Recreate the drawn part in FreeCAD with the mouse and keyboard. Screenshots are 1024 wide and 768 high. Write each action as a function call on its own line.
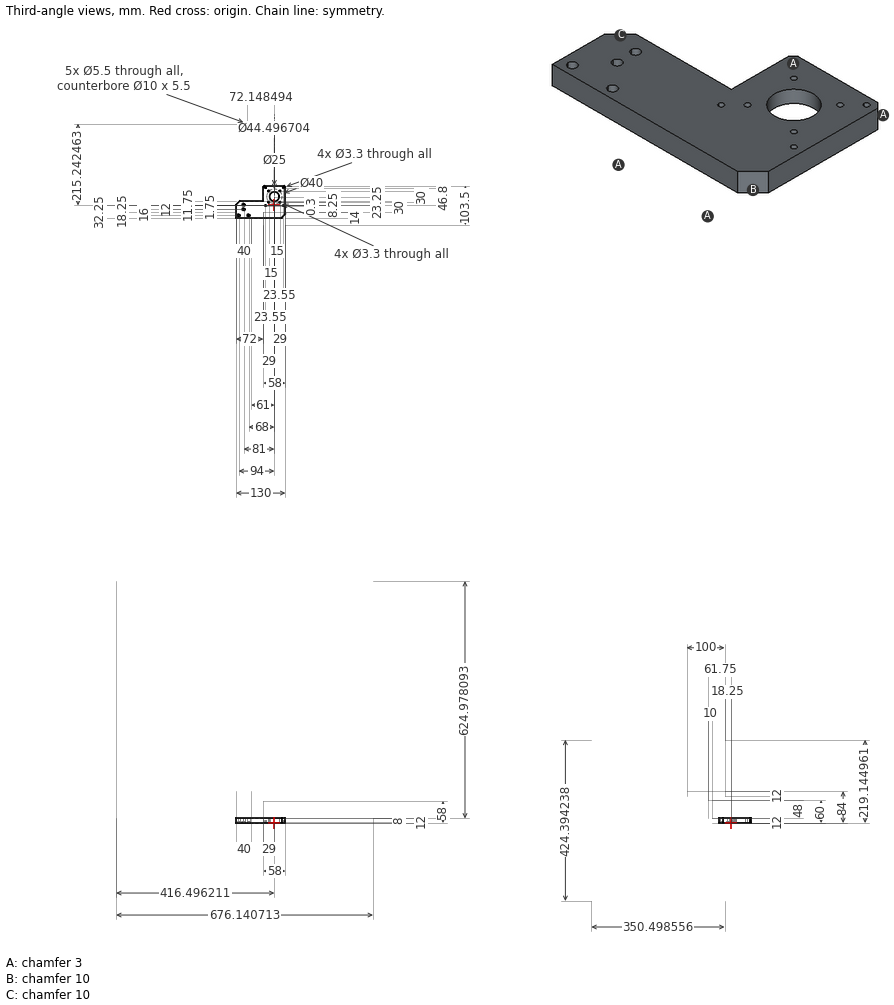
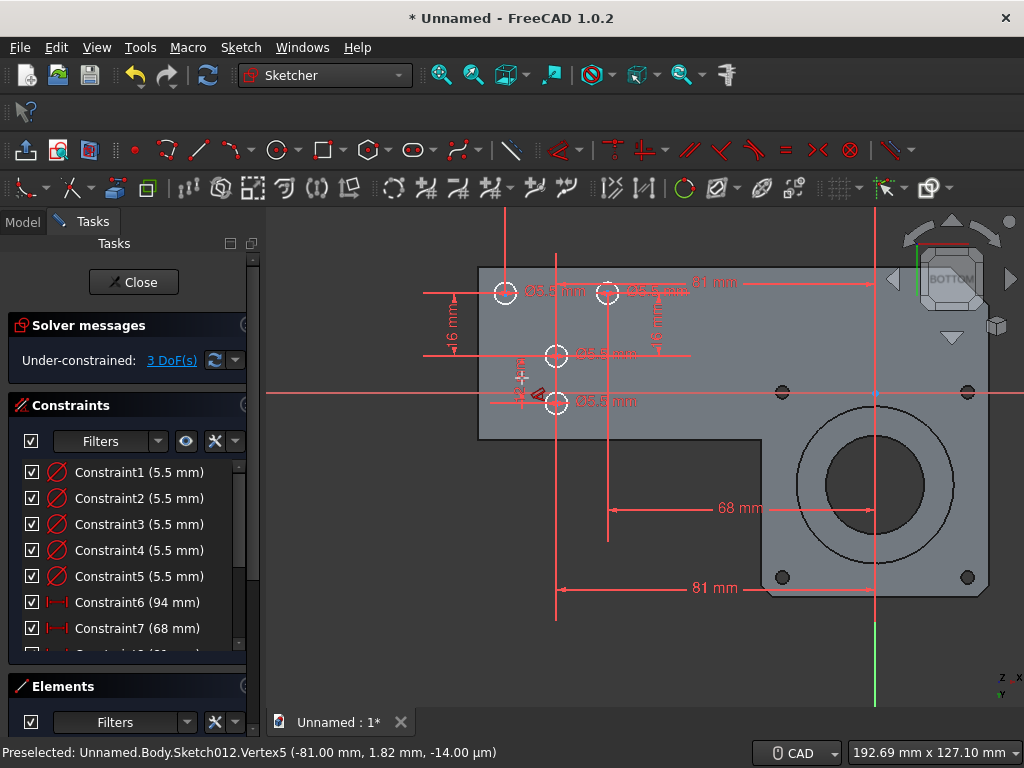
scroll(556, 403, up, 9)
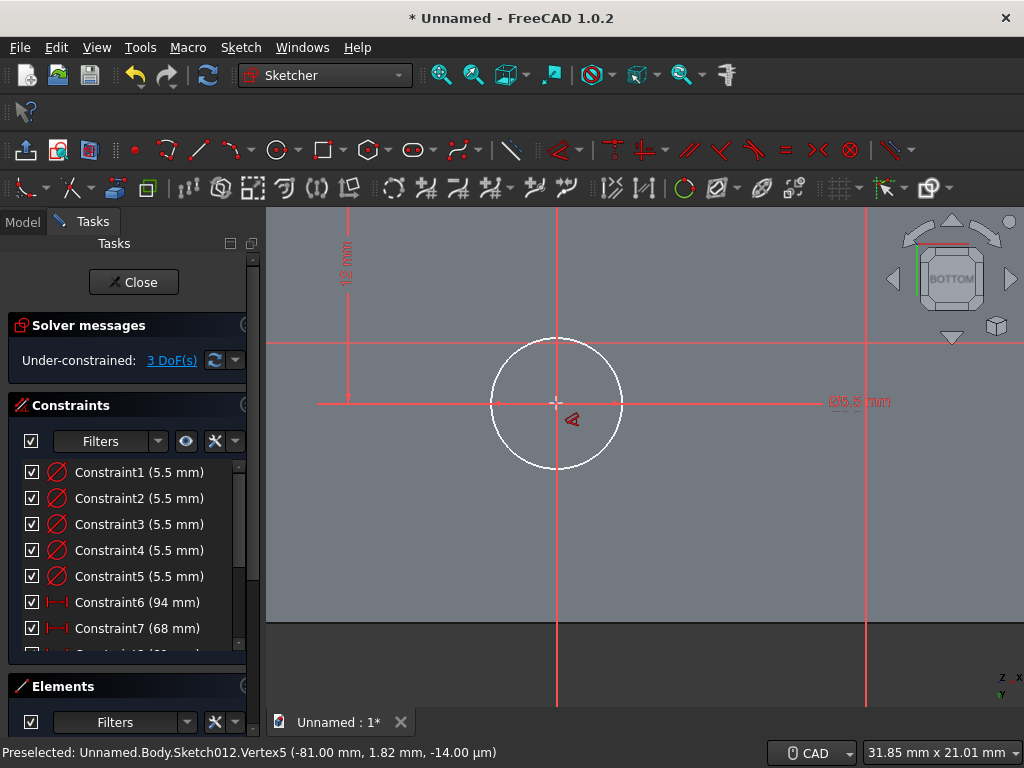
click(557, 404)
click(523, 373)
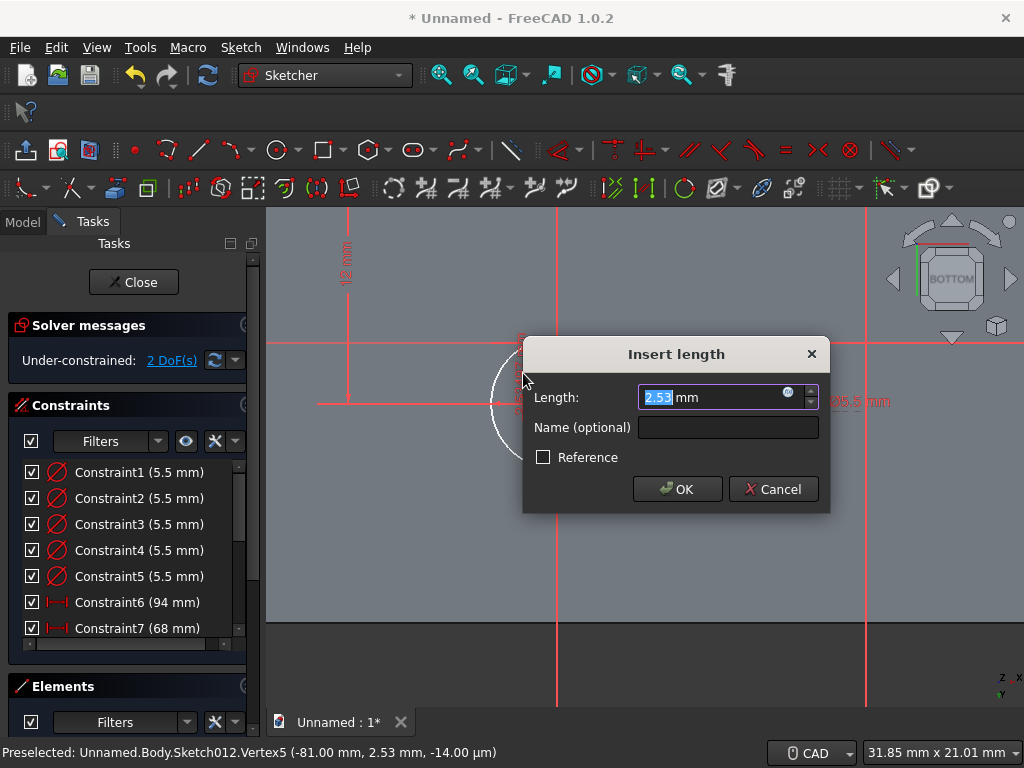
text(1.75)
key(Return)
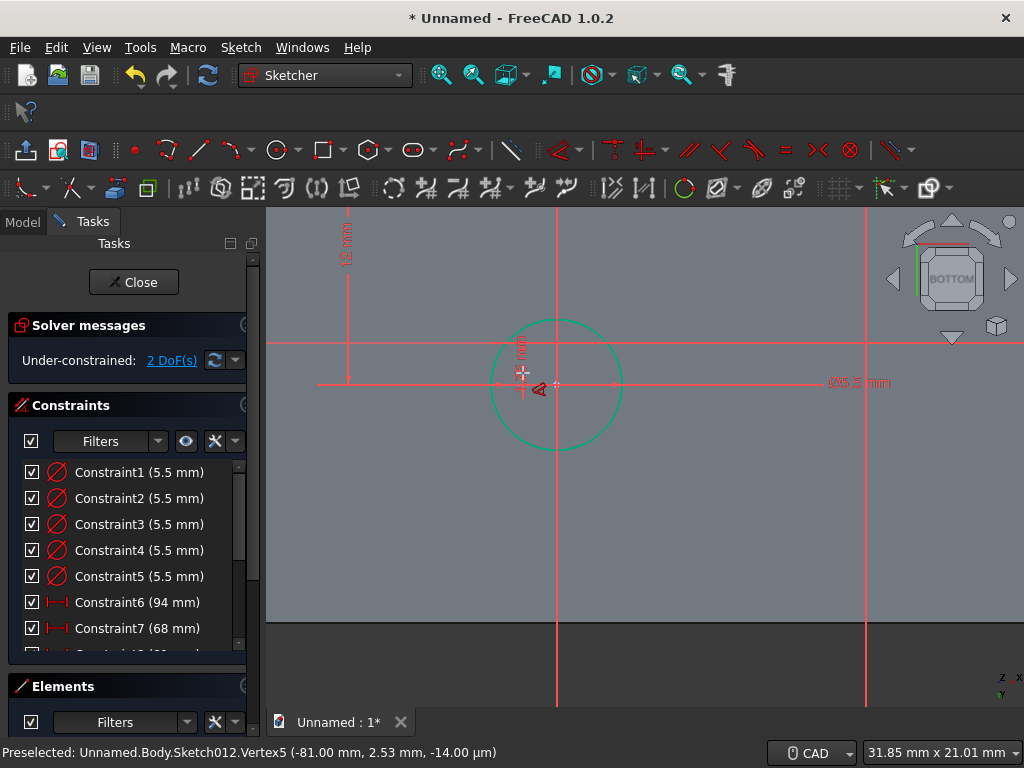
scroll(537, 345, down, 15)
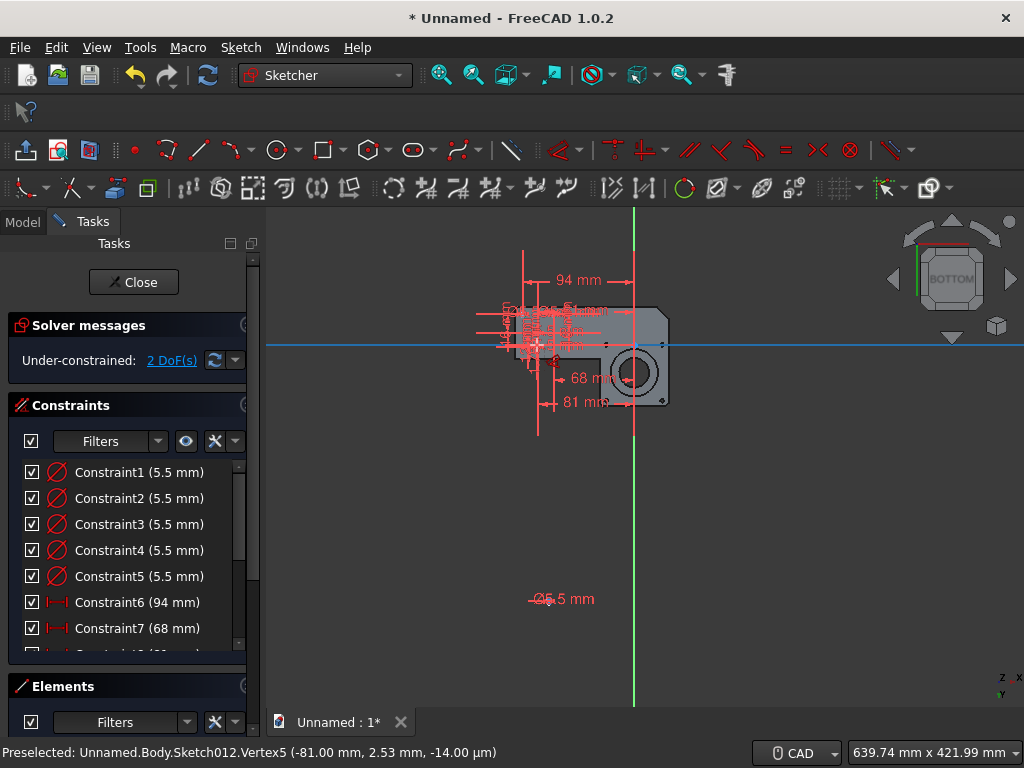
click(549, 601)
click(592, 635)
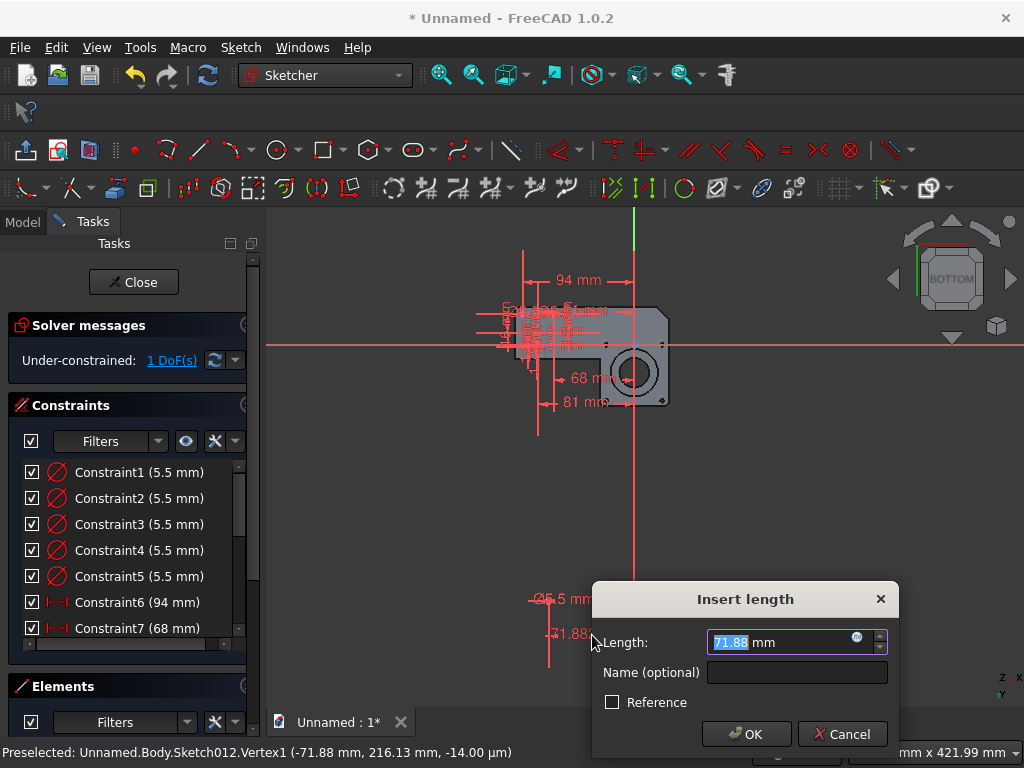
text(72.148494)
key(Return)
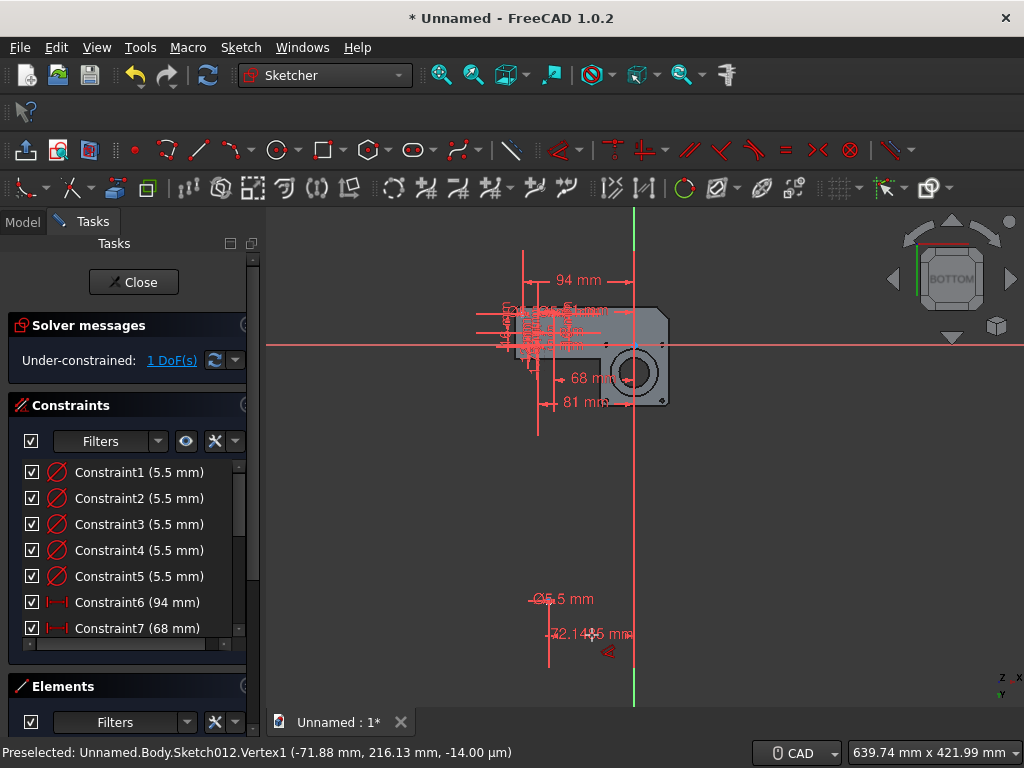
click(549, 601)
click(668, 473)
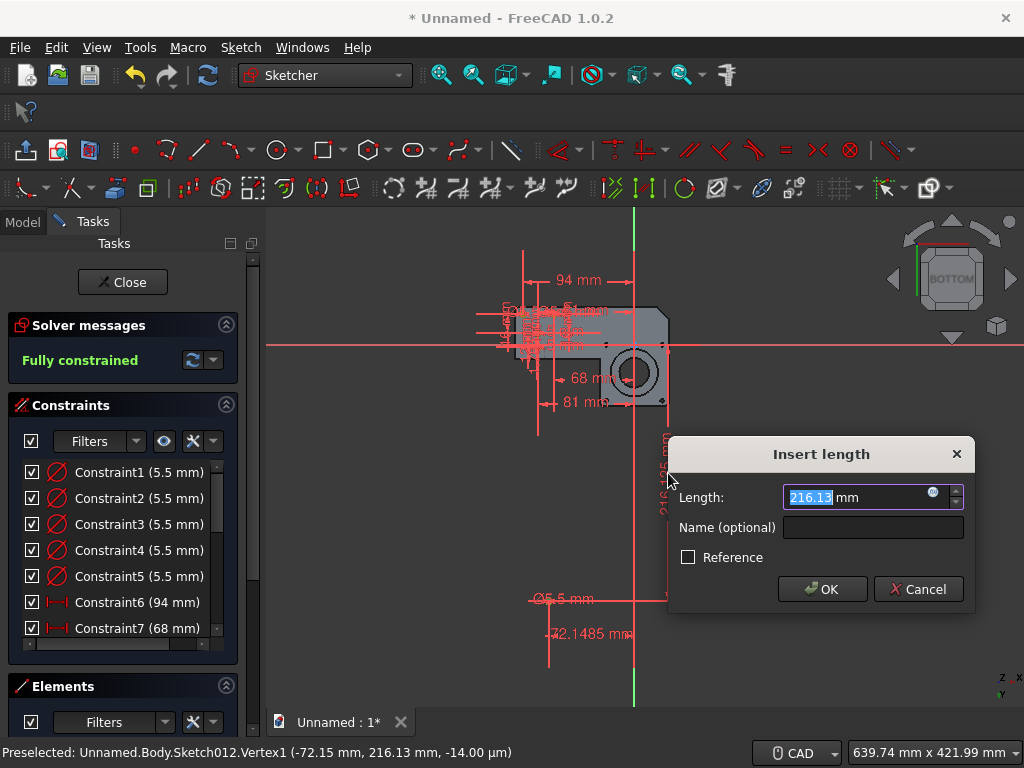
text(215.242463)
key(Return)
key(Escape)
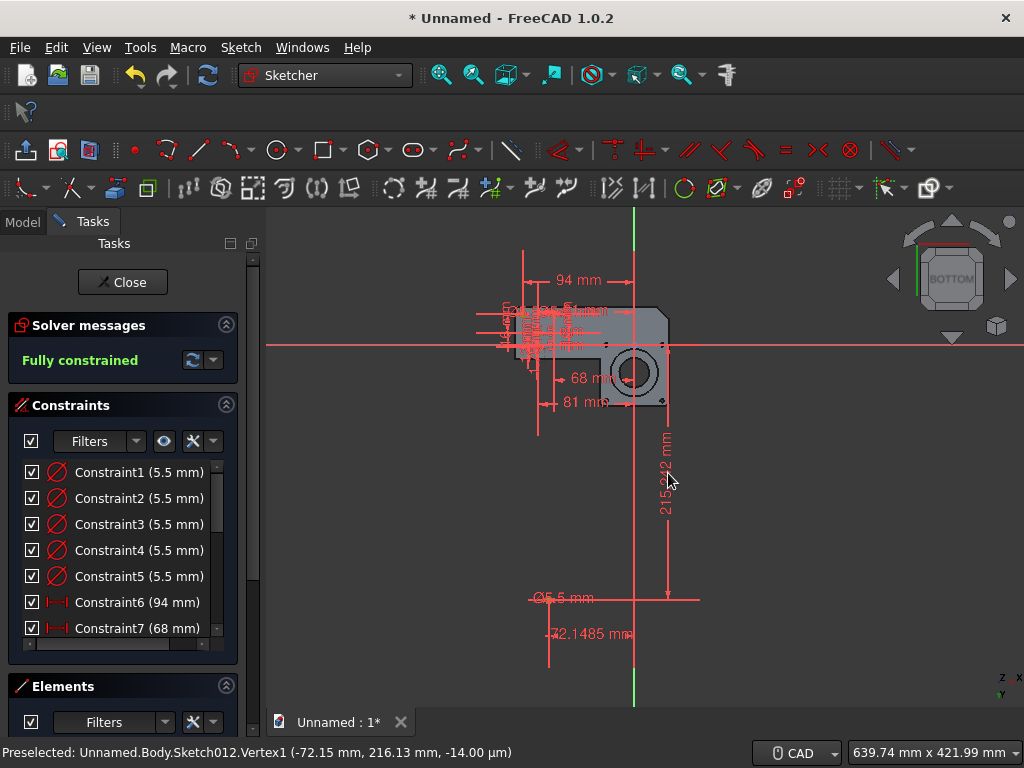
click(123, 282)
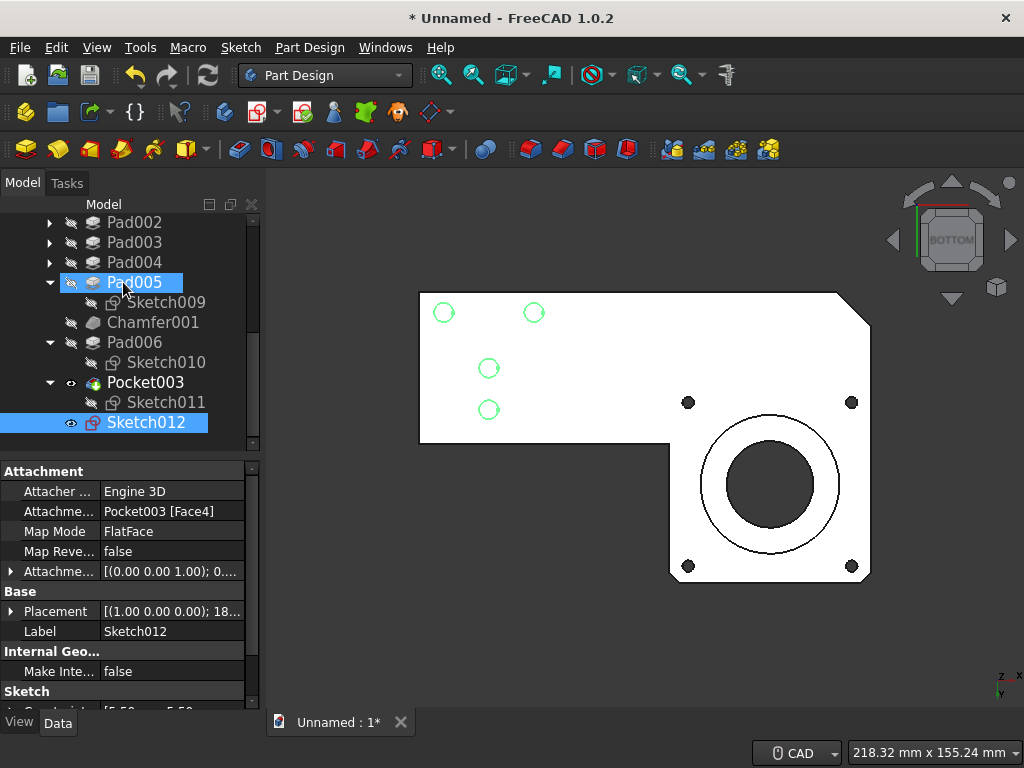
click(272, 150)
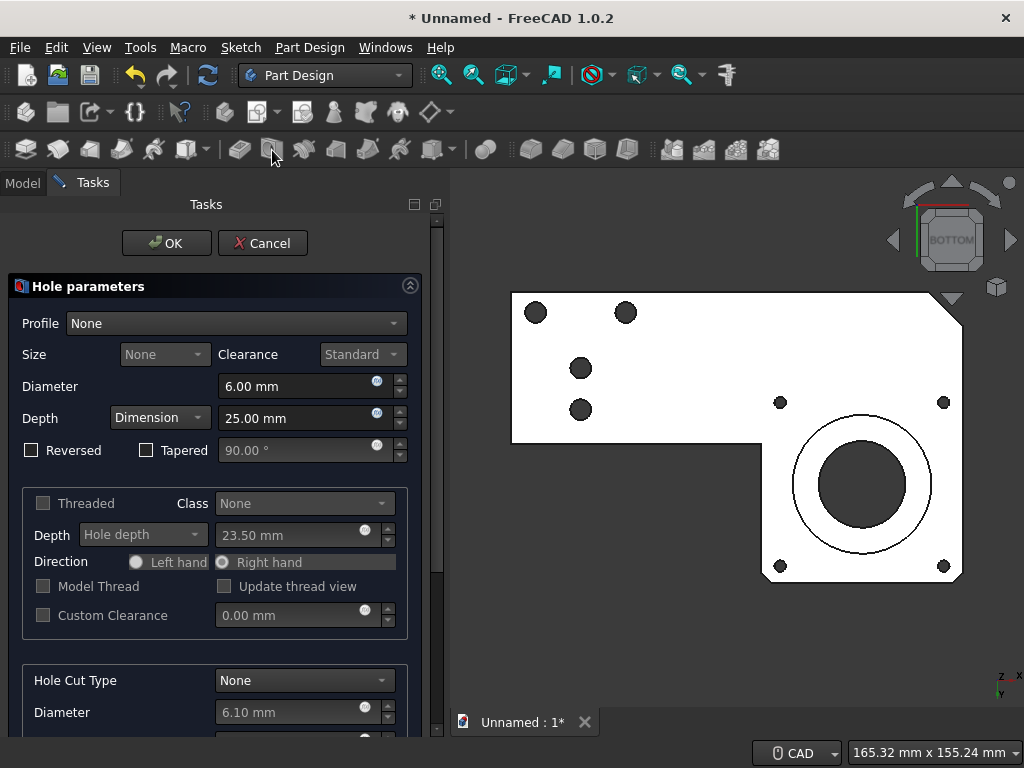
triple_click(305, 386)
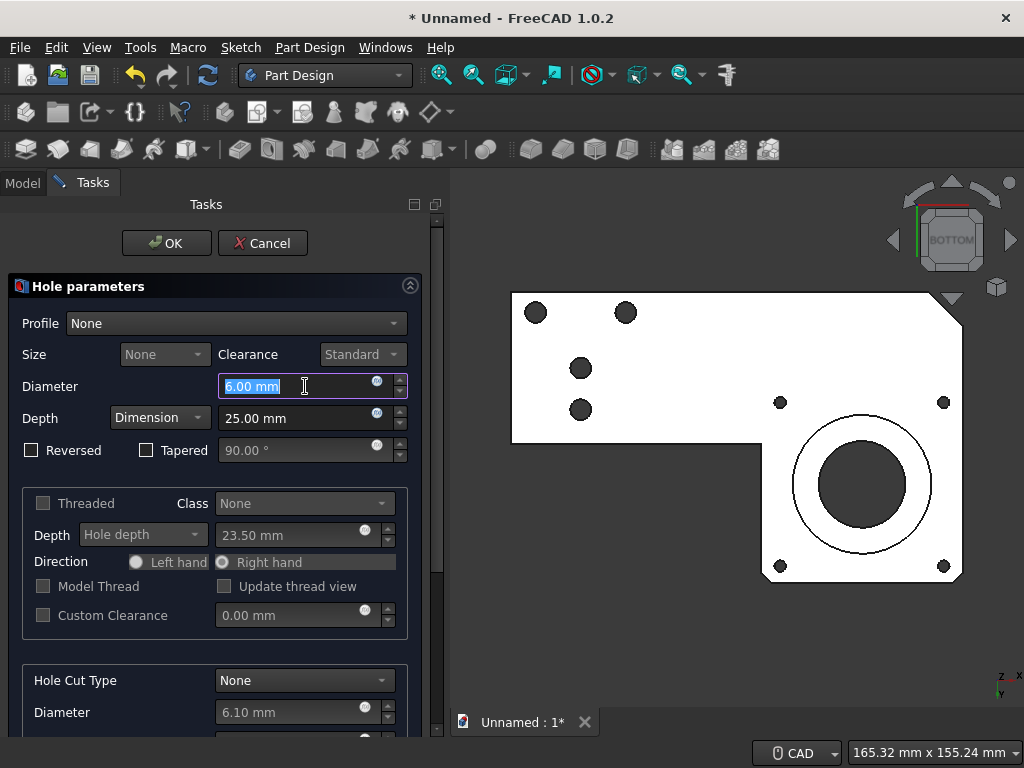
text(5.5)
key(Tab)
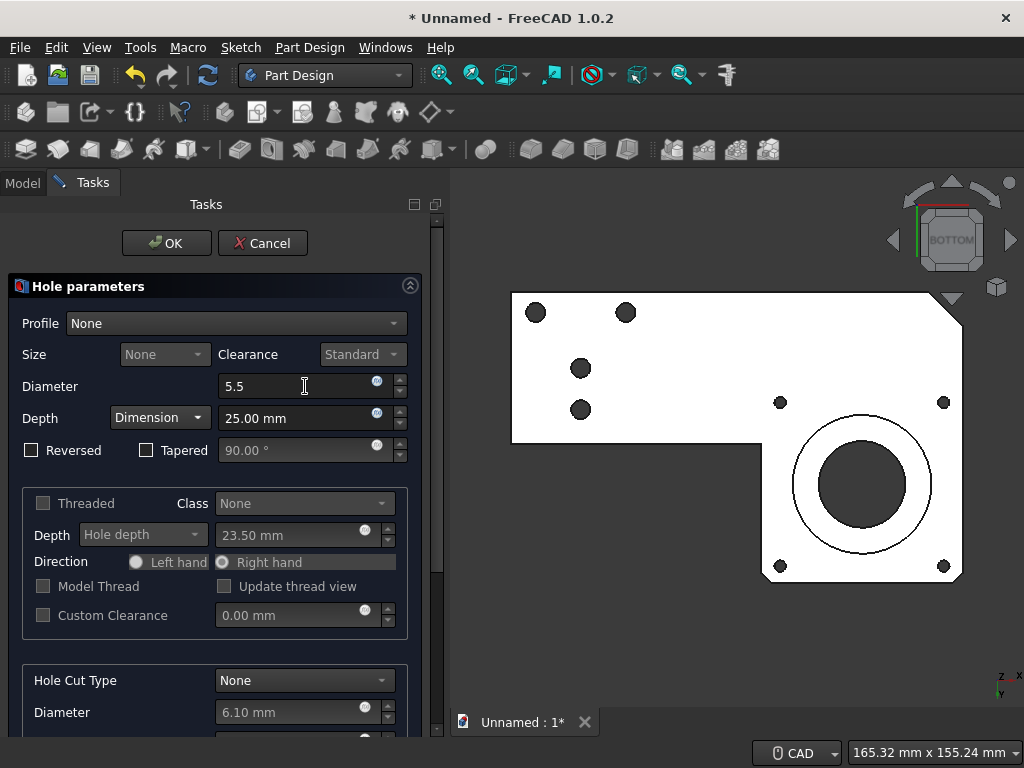
click(161, 418)